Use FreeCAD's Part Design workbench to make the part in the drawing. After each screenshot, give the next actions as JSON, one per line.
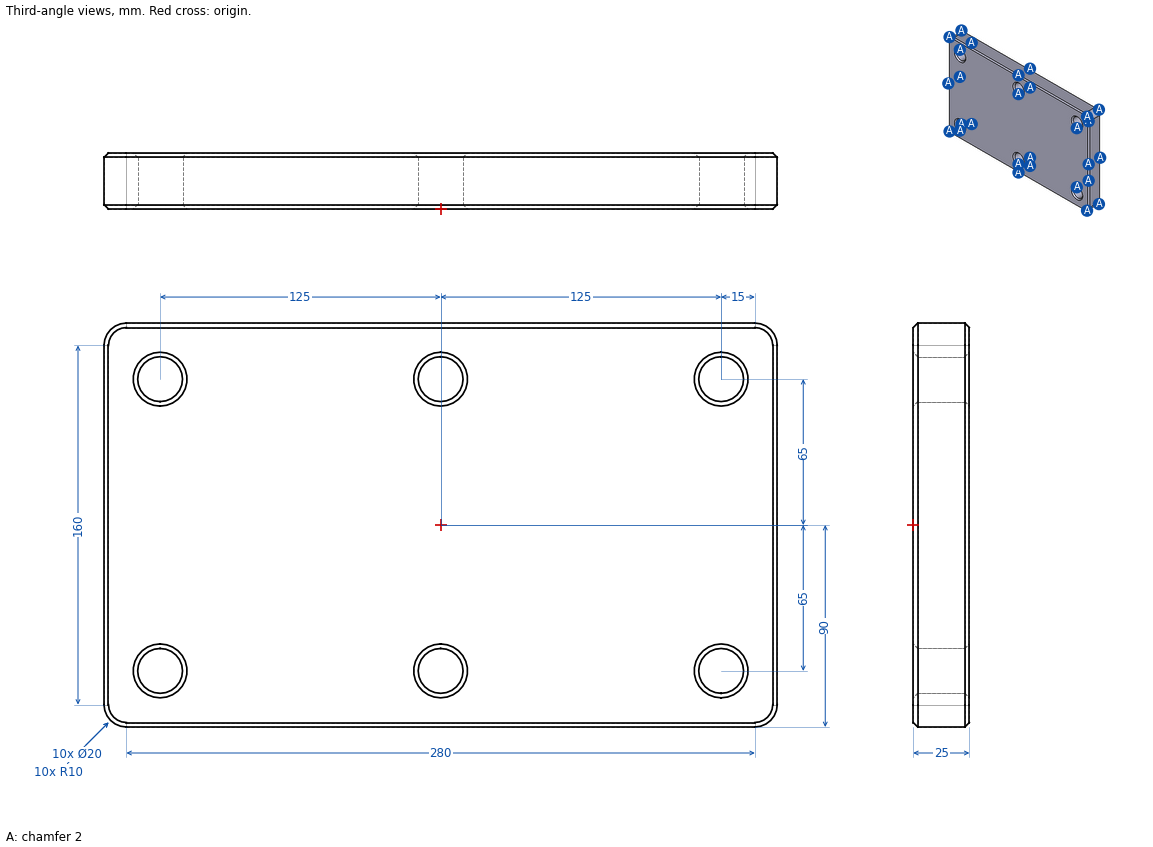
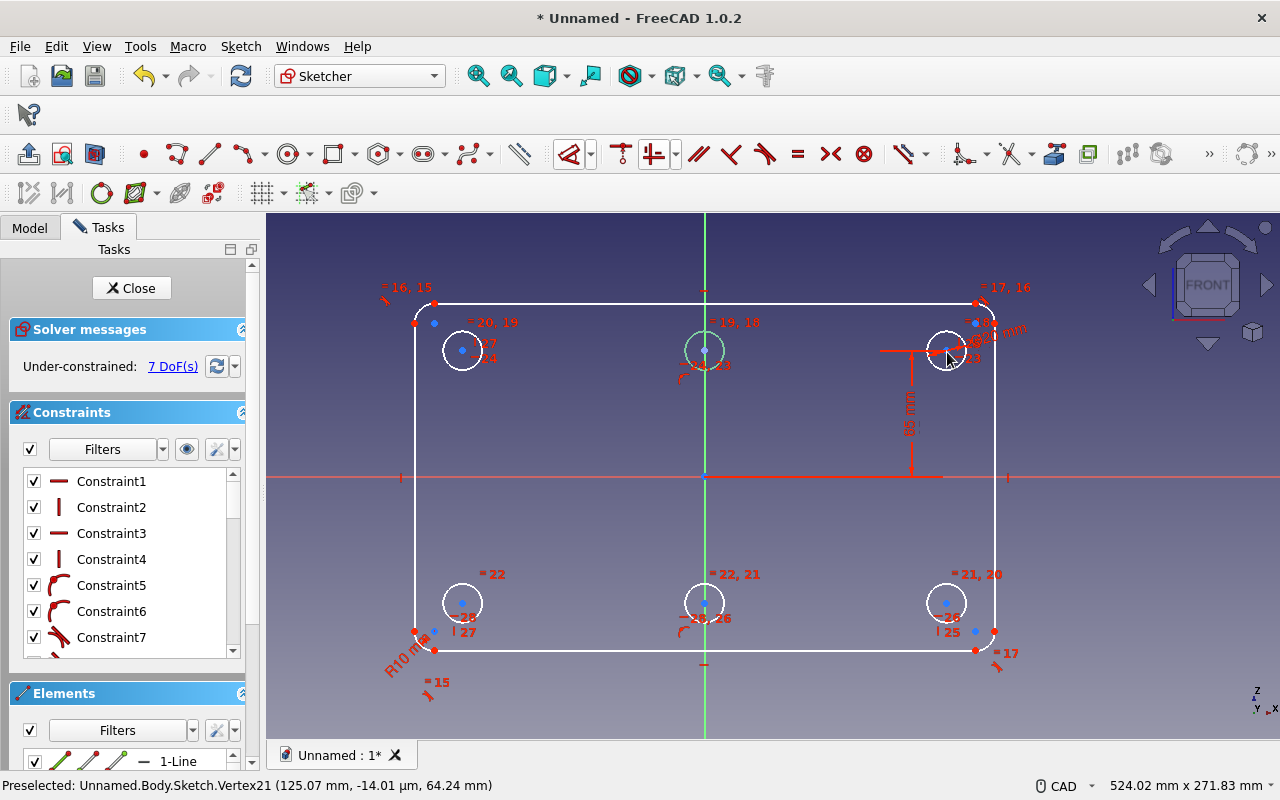
{"action": "left_click", "coordinate": [947, 603]}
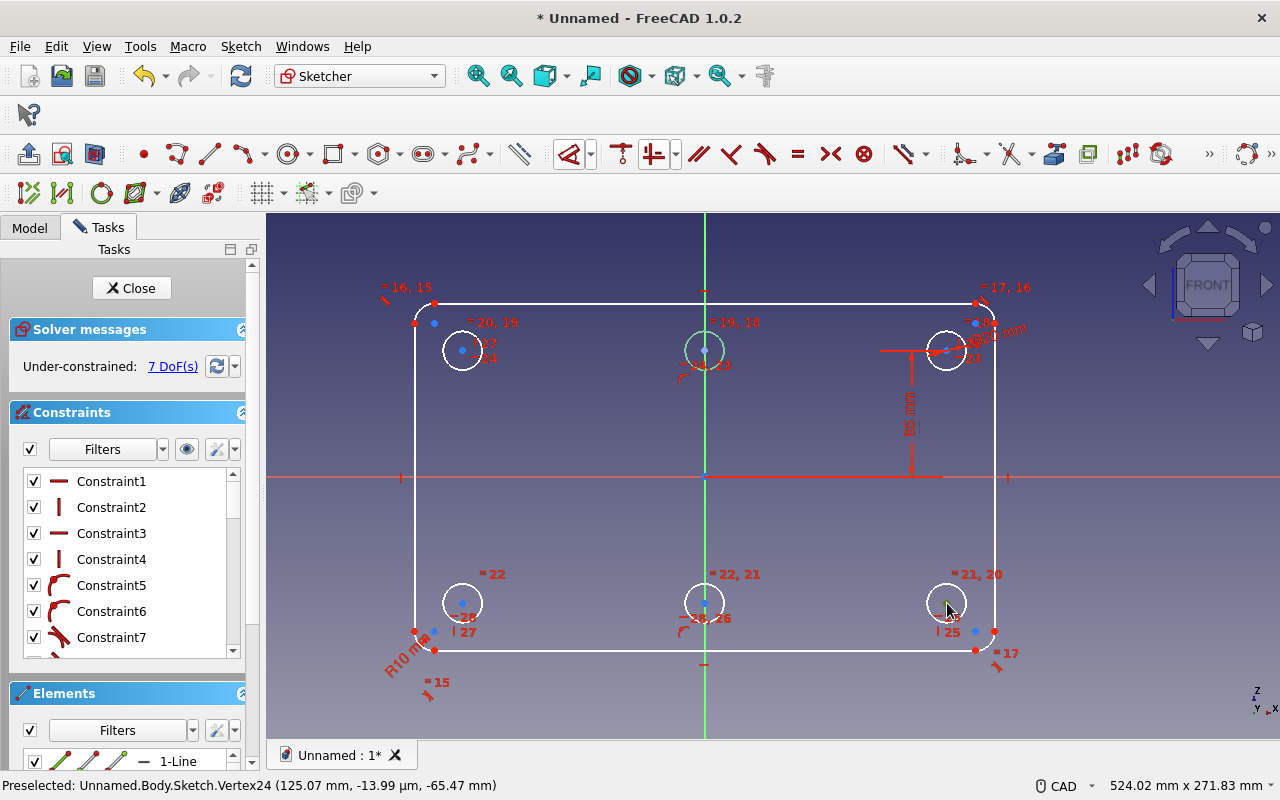
{"action": "key", "text": "i"}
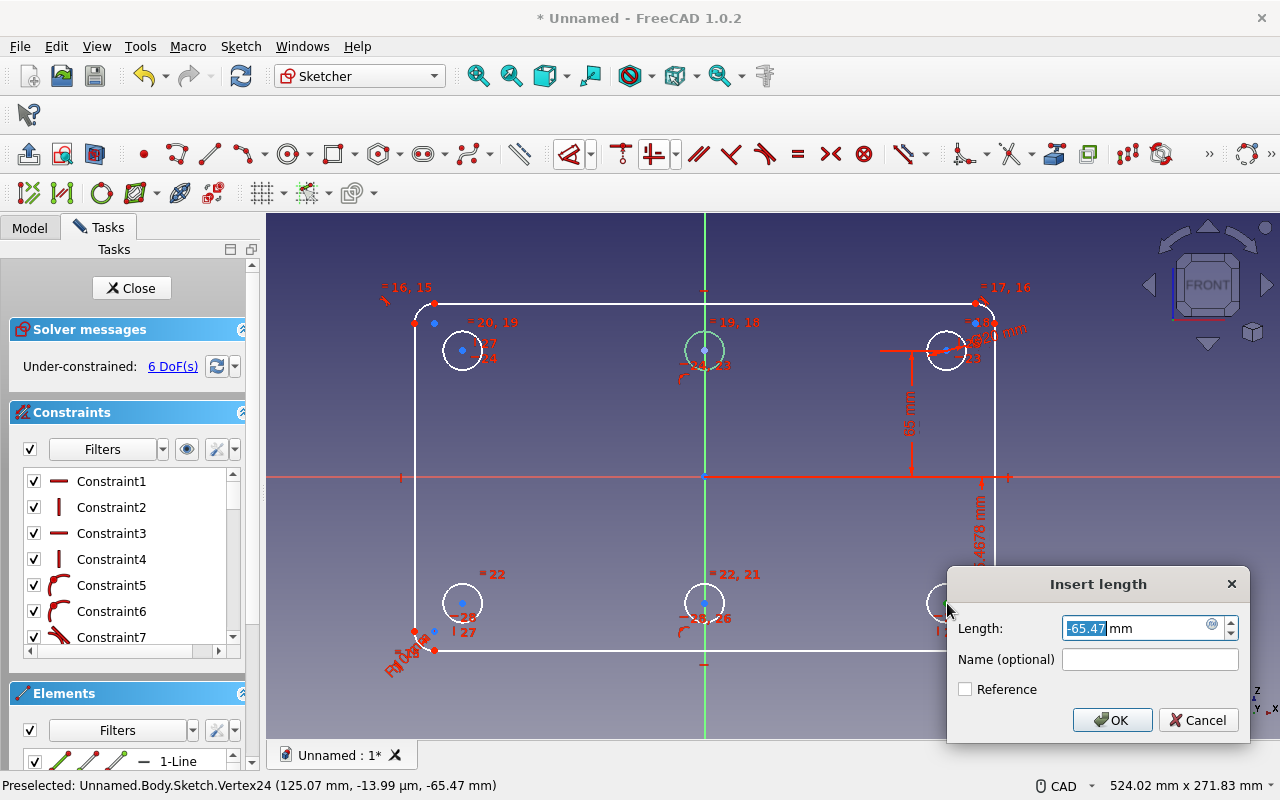
{"action": "type", "text": "-65"}
{"action": "key", "text": "Return"}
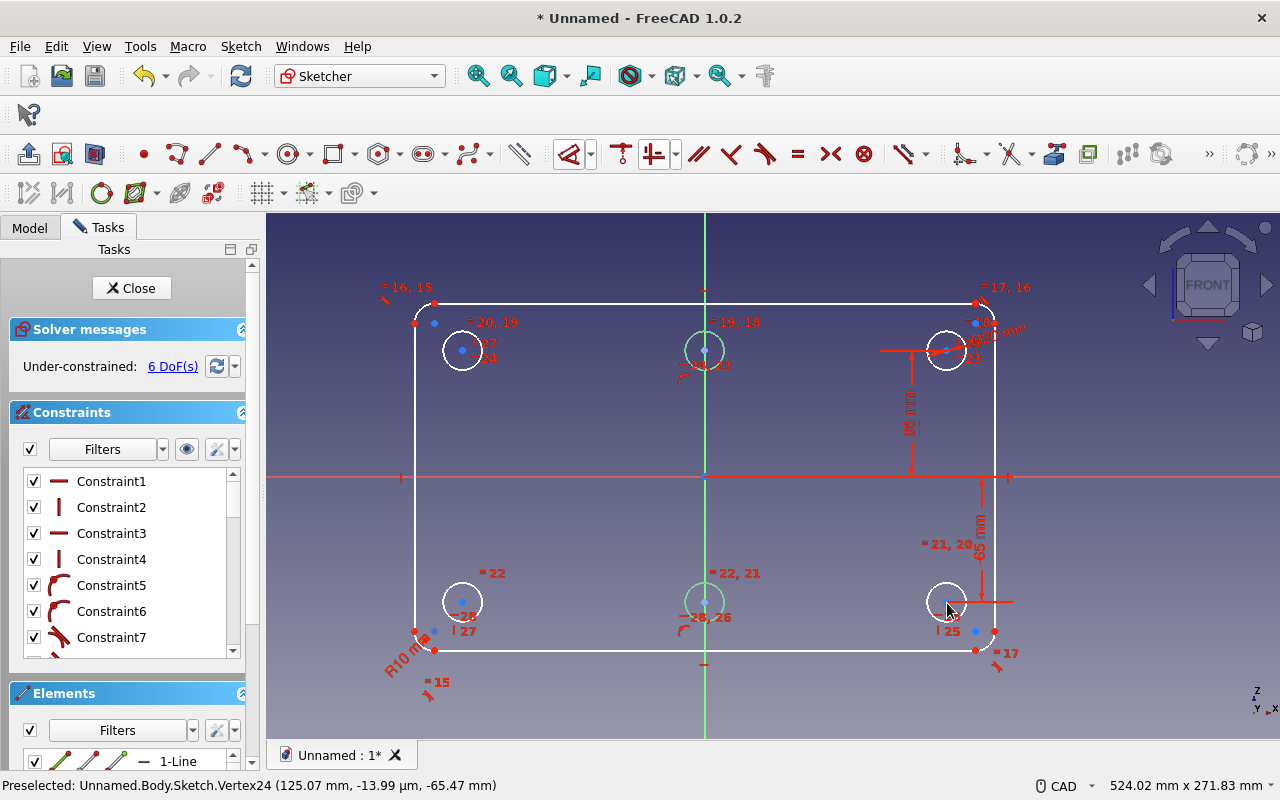
{"action": "left_click", "coordinate": [813, 651]}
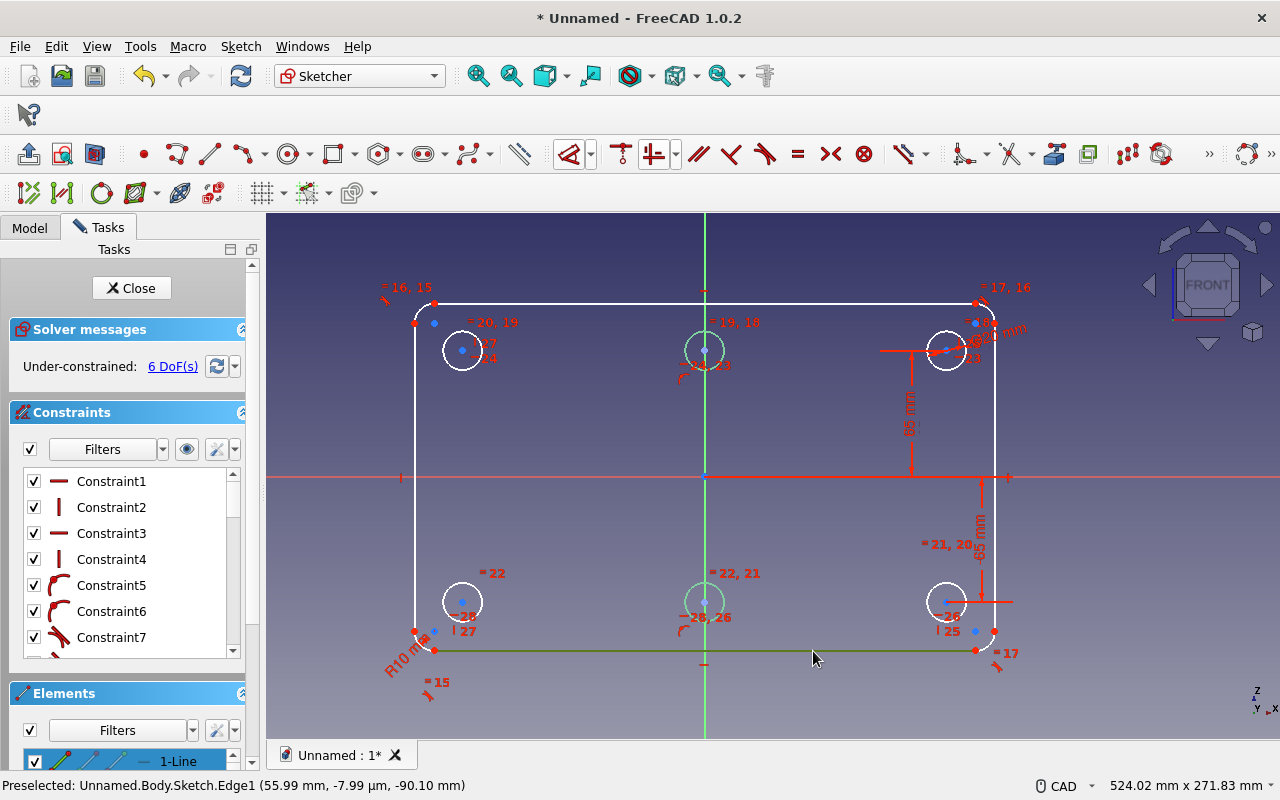
{"action": "key", "text": "l"}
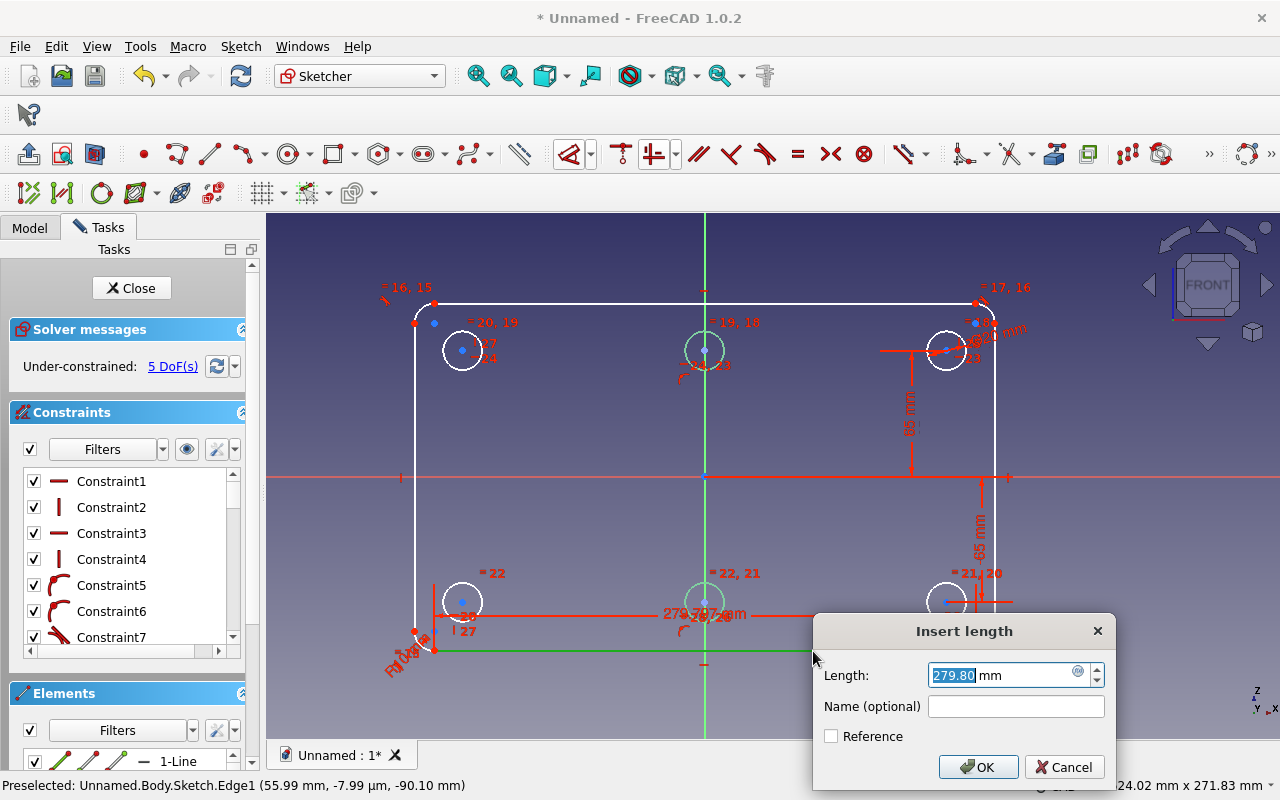
{"action": "type", "text": "280"}
{"action": "key", "text": "Return"}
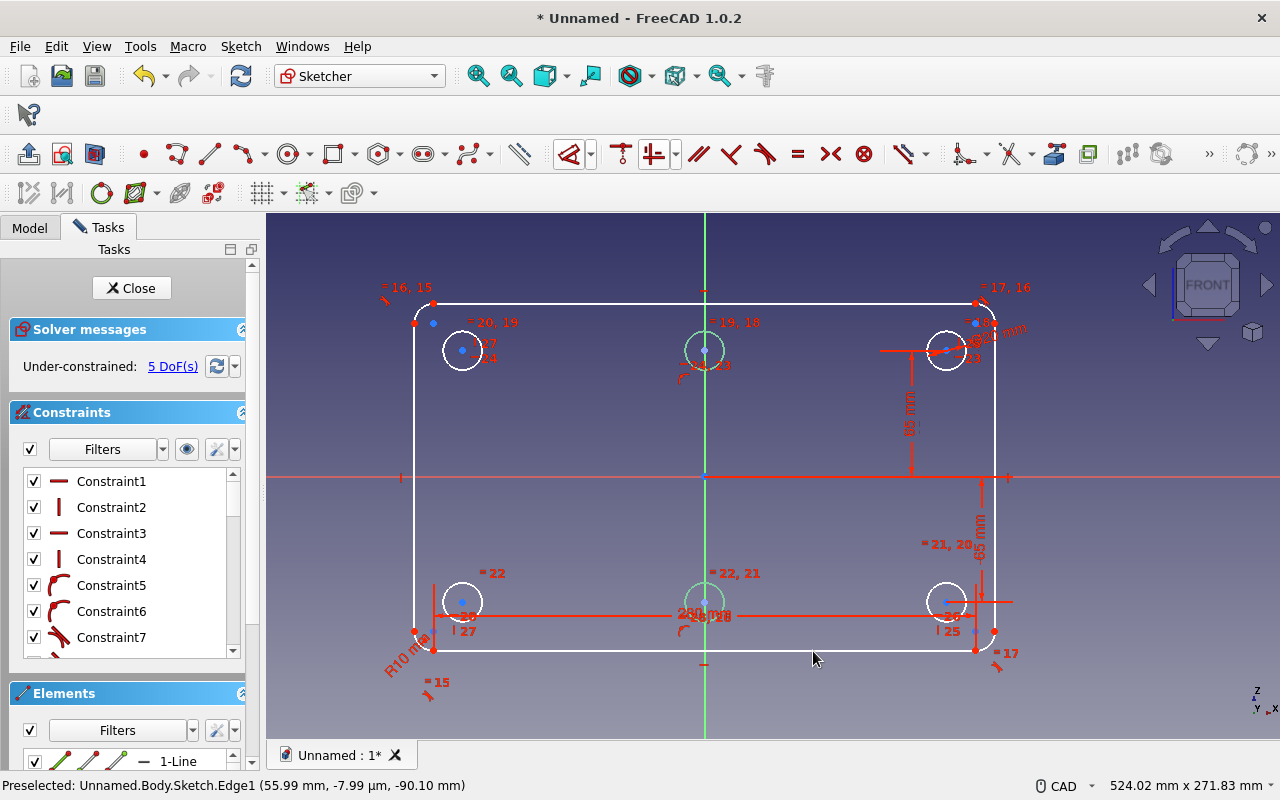
{"action": "left_click", "coordinate": [414, 539]}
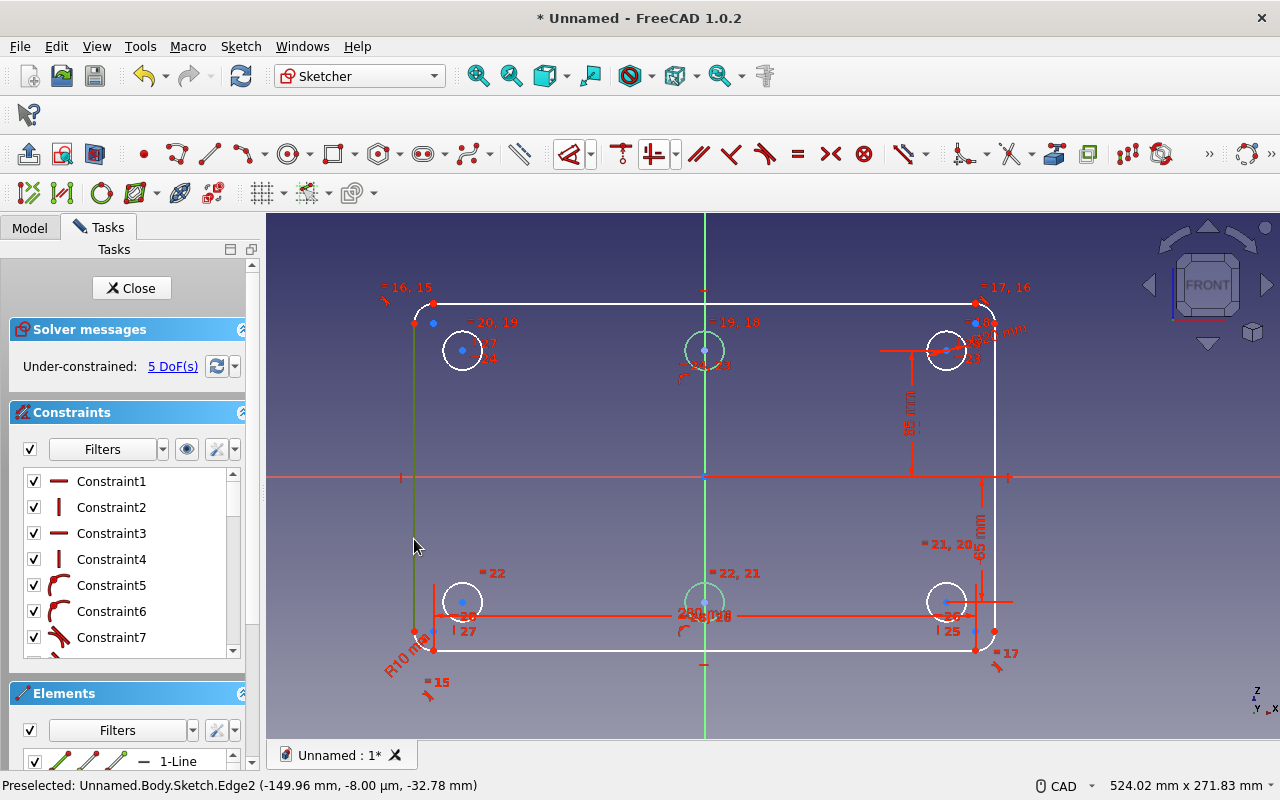
{"action": "left_click", "coordinate": [590, 154]}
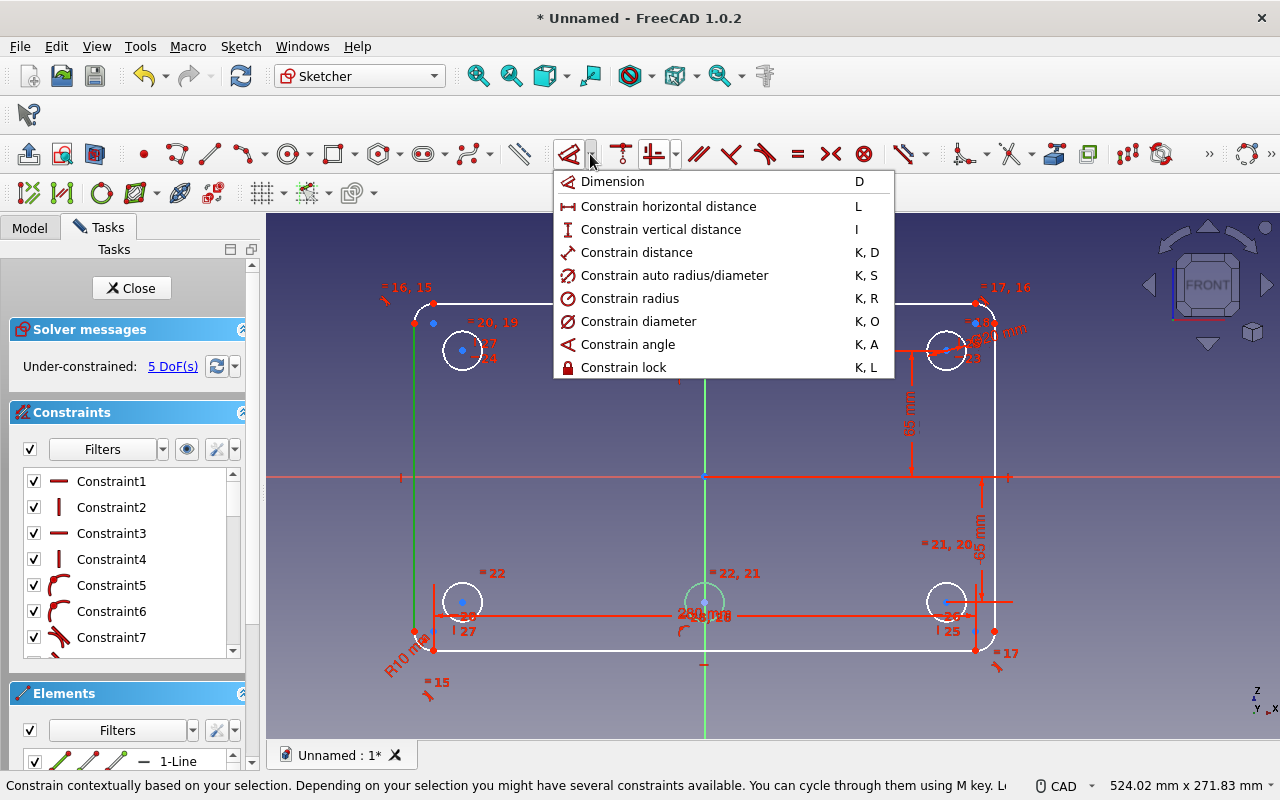
{"action": "left_click", "coordinate": [724, 230]}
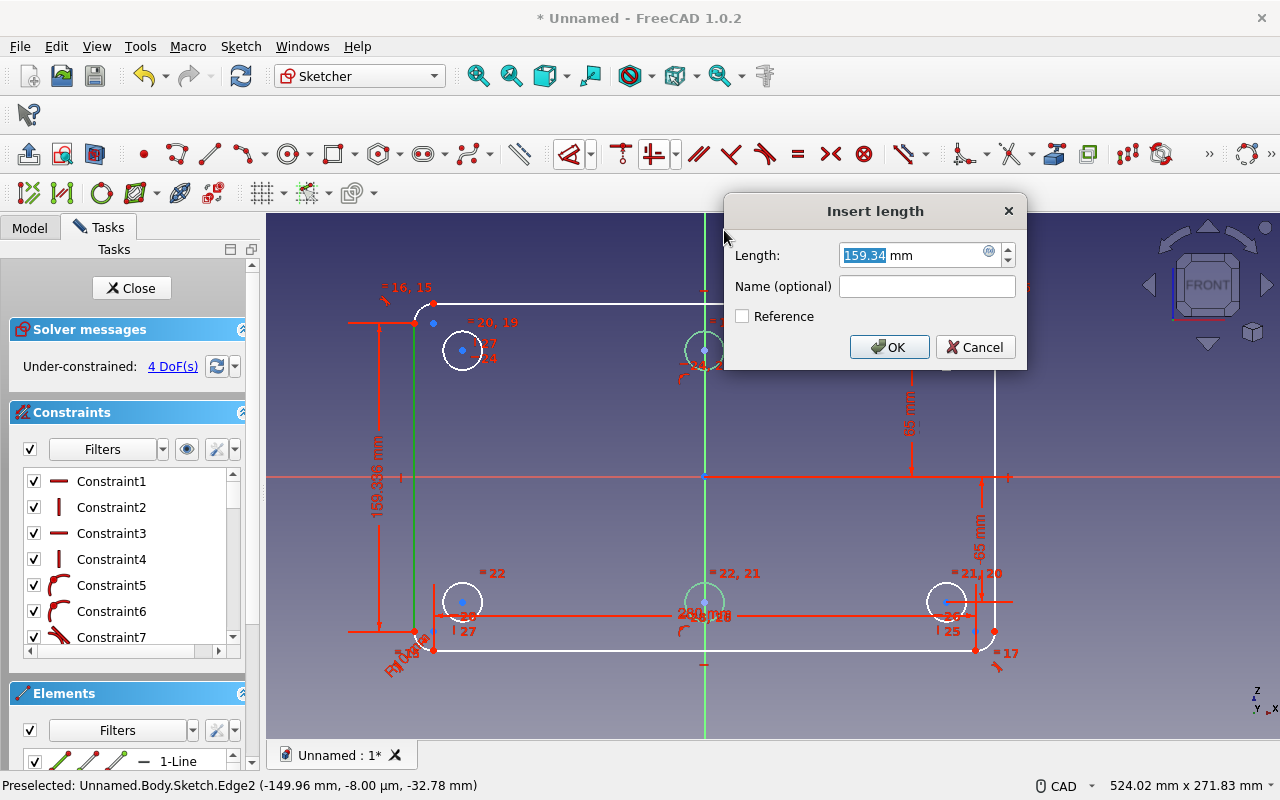
{"action": "type", "text": "160"}
{"action": "key", "text": "Return"}